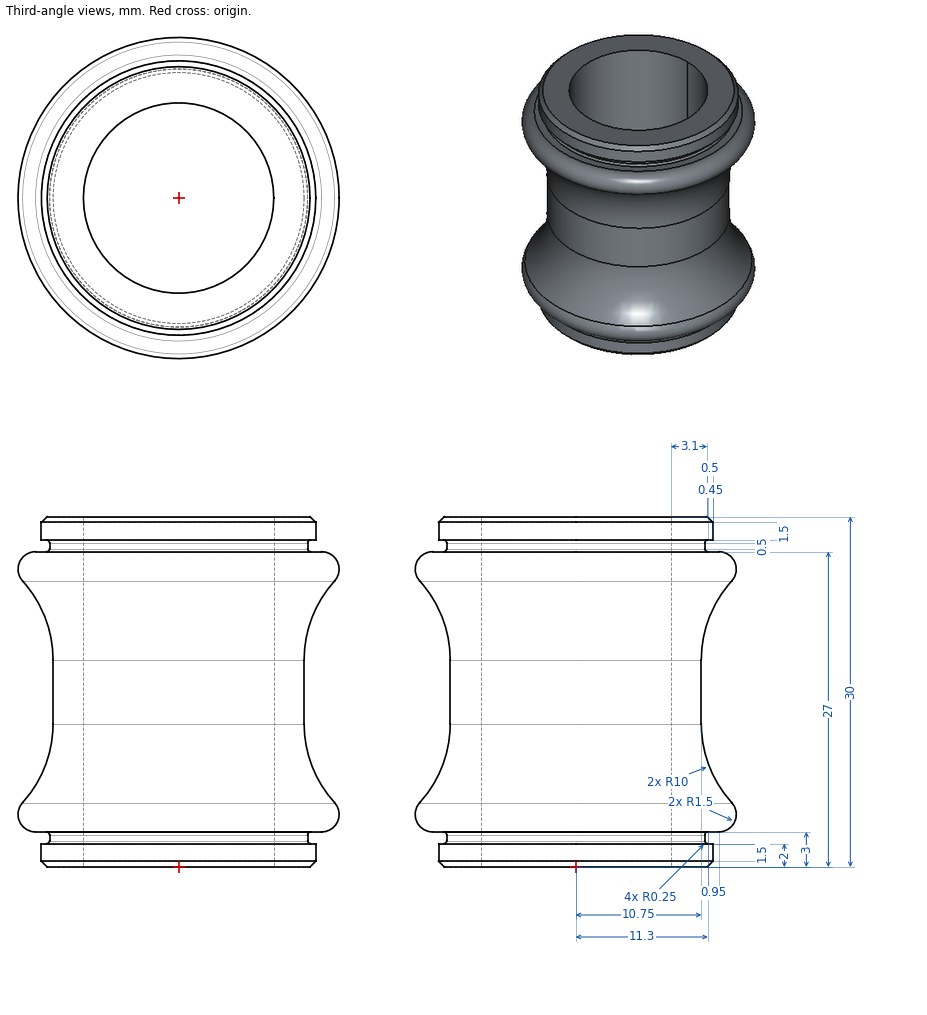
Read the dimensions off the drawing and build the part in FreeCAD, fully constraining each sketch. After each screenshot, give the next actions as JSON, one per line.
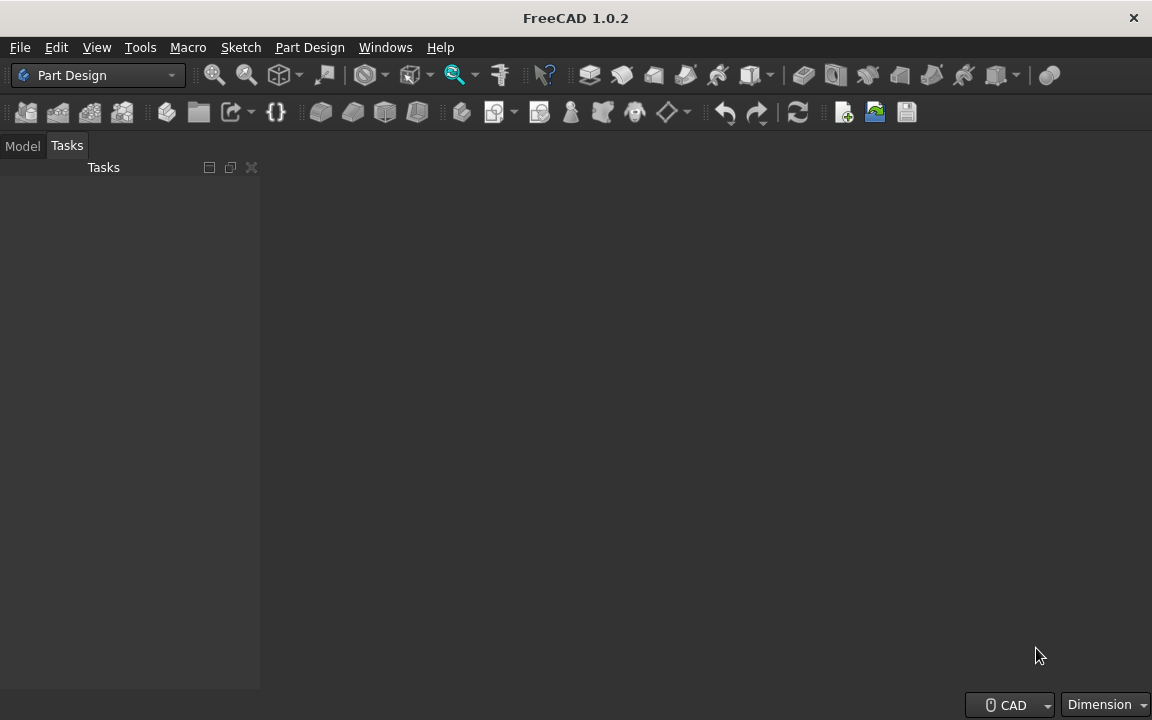
{"action": "left_click", "coordinate": [844, 112]}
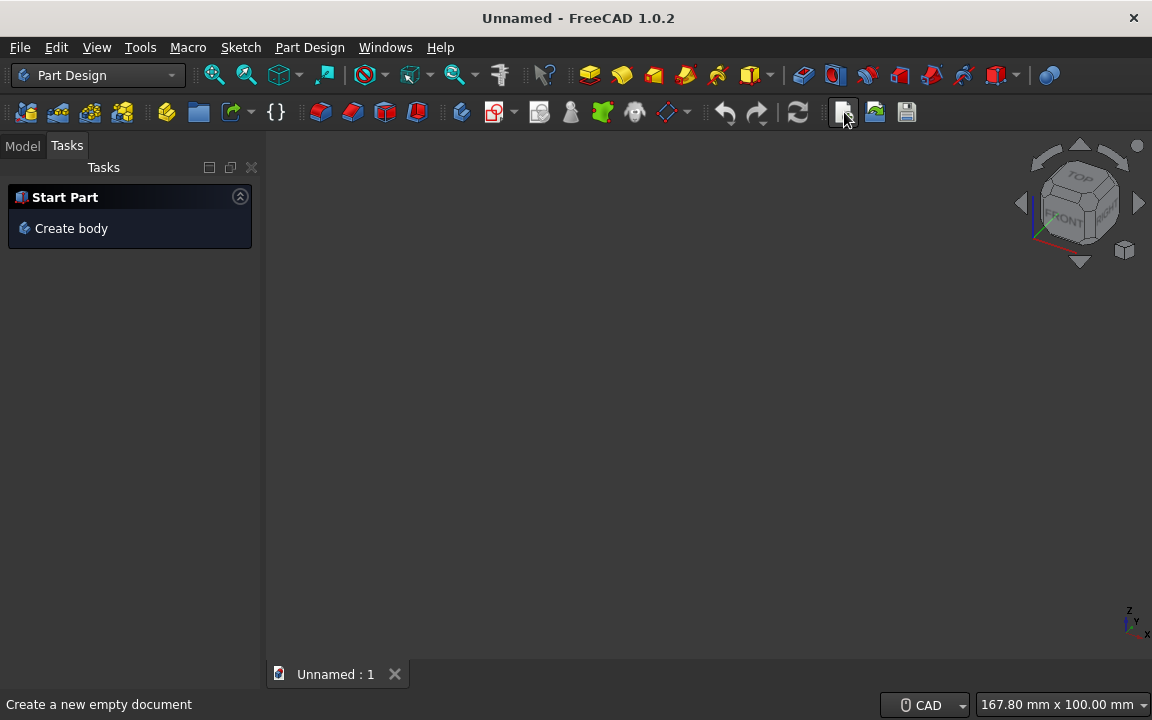
{"action": "left_click", "coordinate": [494, 112]}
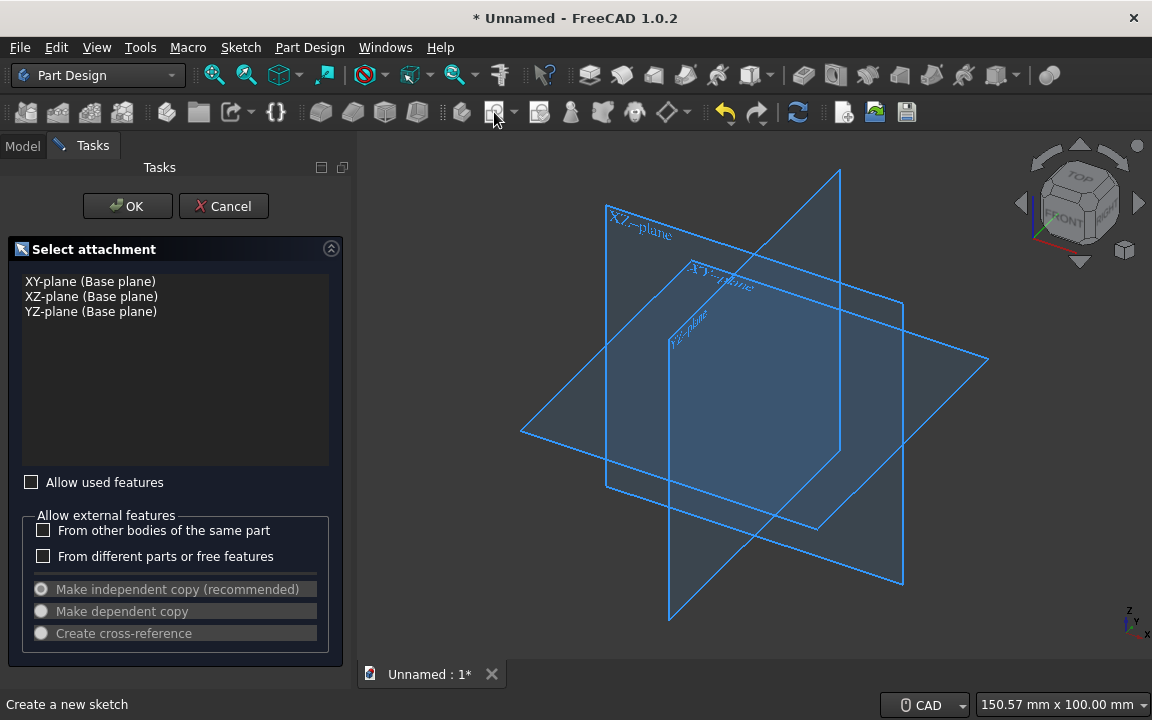
{"action": "left_click", "coordinate": [82, 312]}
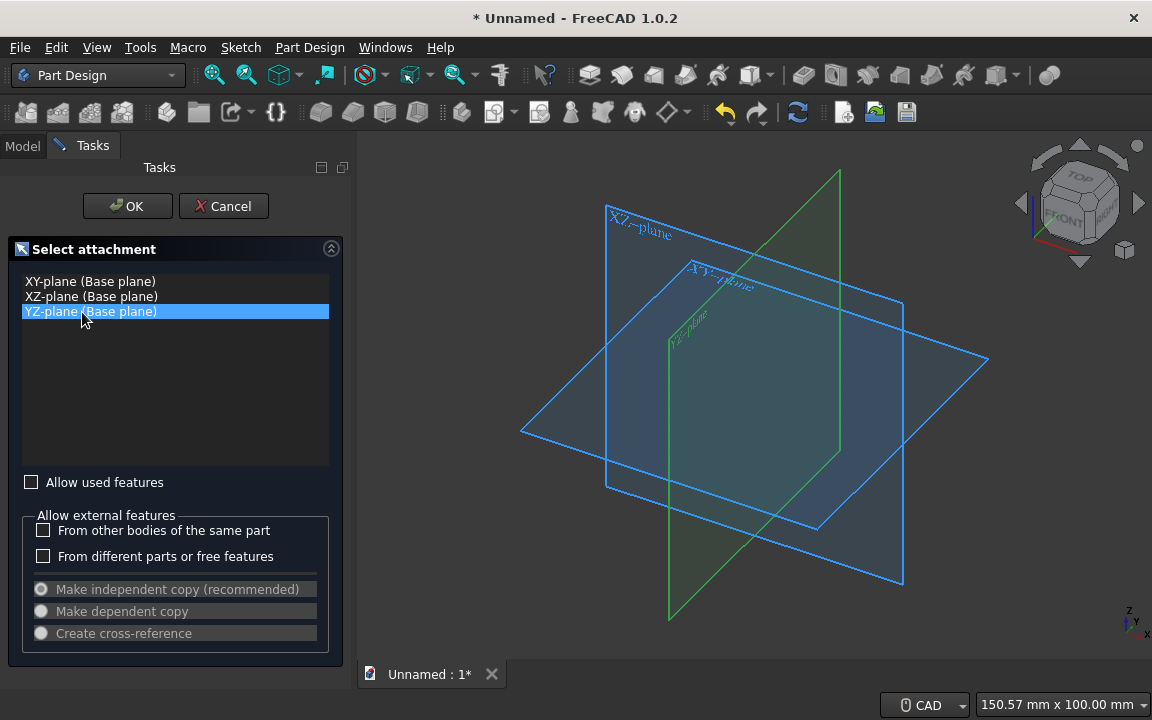
{"action": "left_click", "coordinate": [128, 206]}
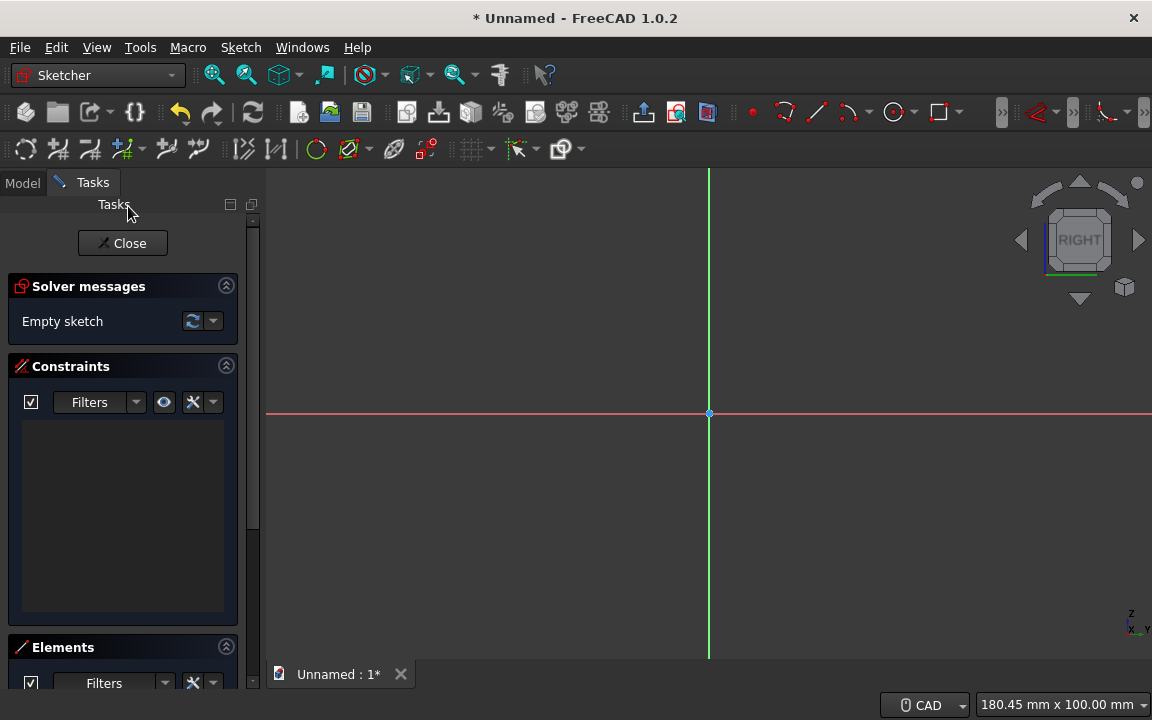
{"action": "scroll", "coordinate": [826, 280], "scroll_direction": "up", "scroll_amount": 4}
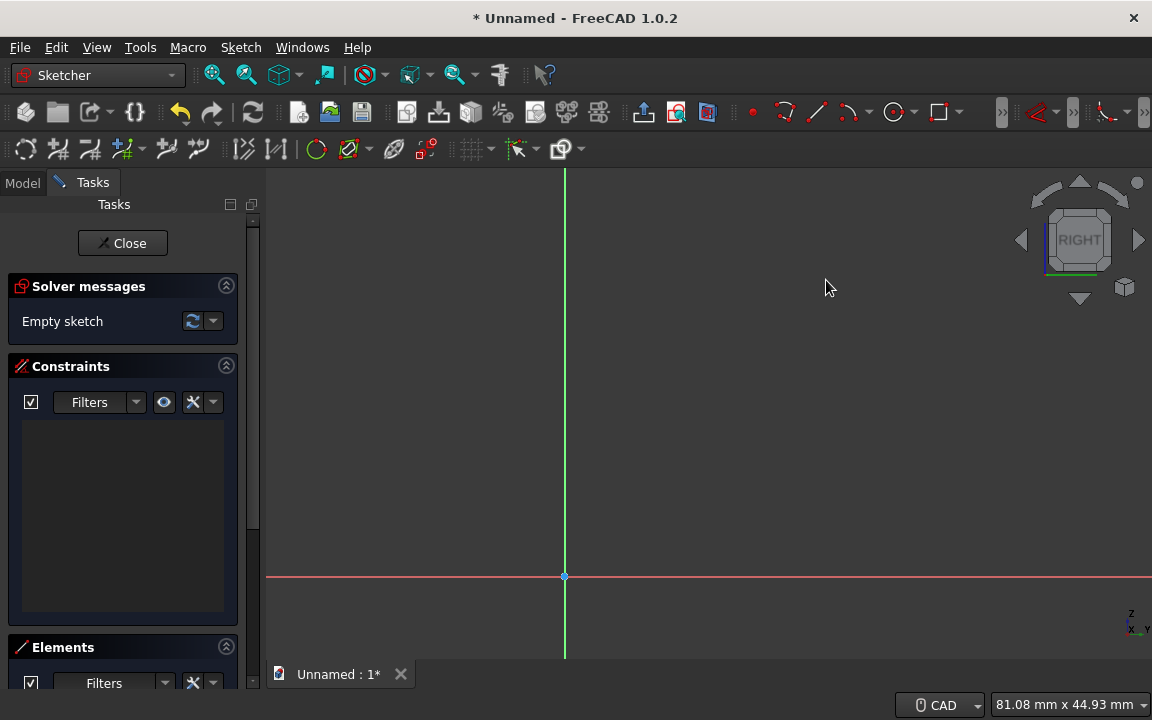
{"action": "left_click", "coordinate": [818, 112]}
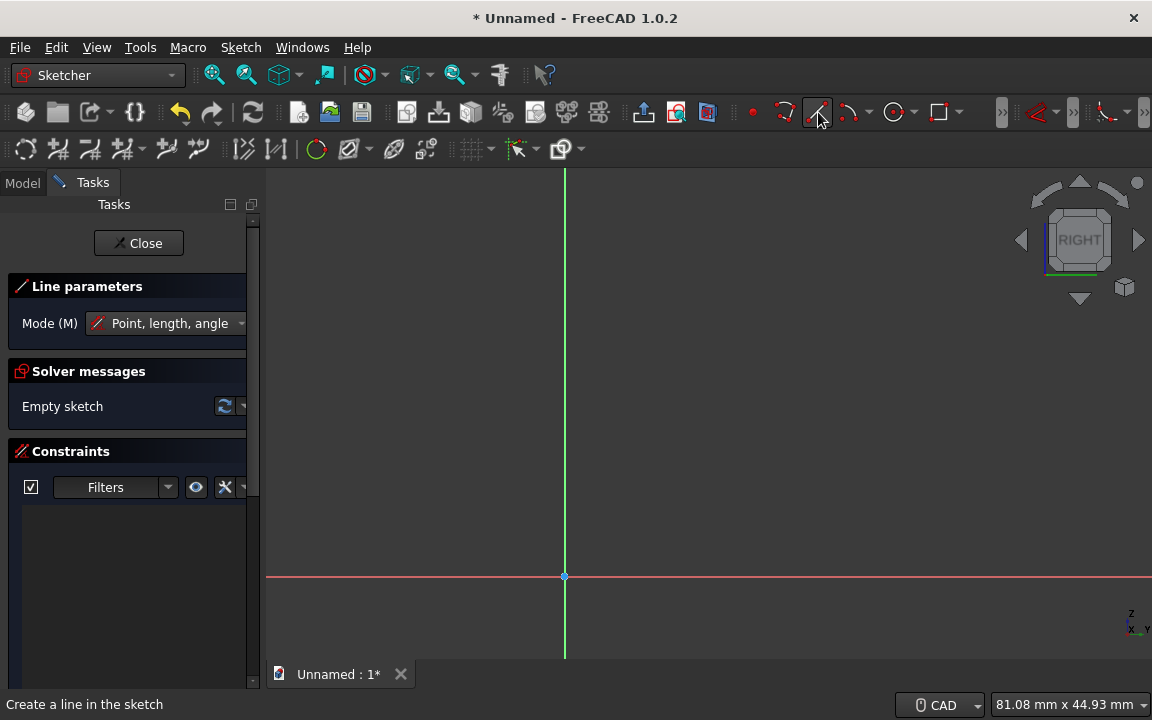
{"action": "left_click", "coordinate": [686, 552]}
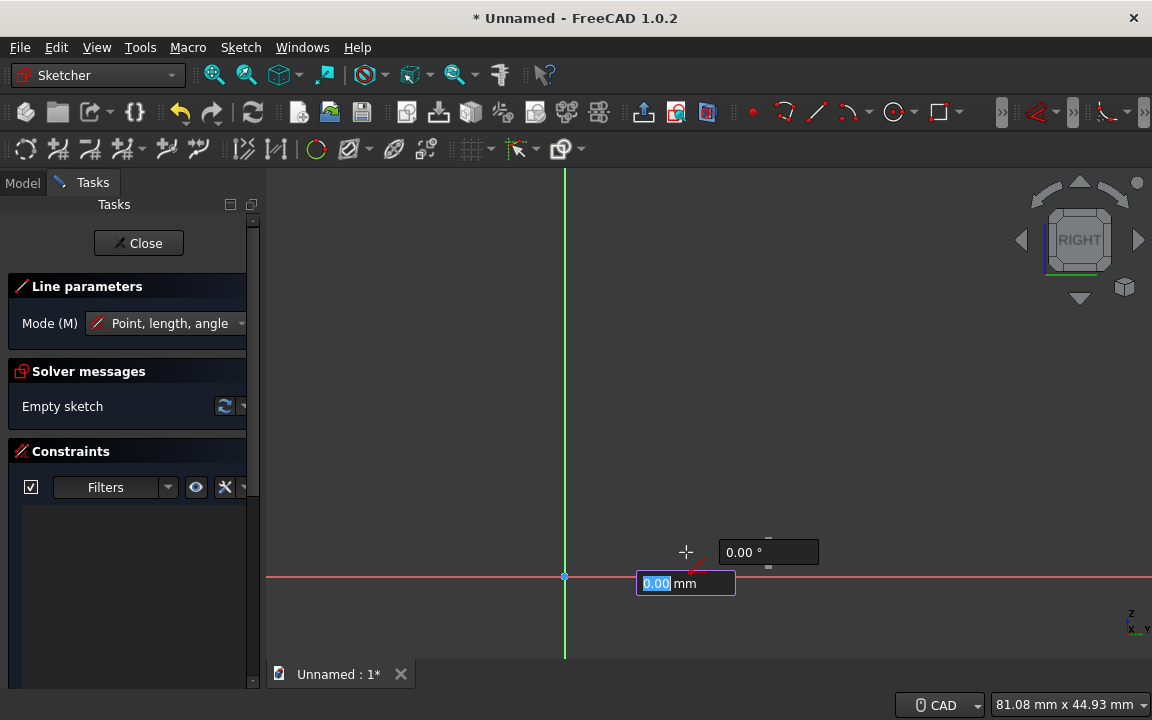
{"action": "scroll", "coordinate": [686, 547], "scroll_direction": "up", "scroll_amount": 6}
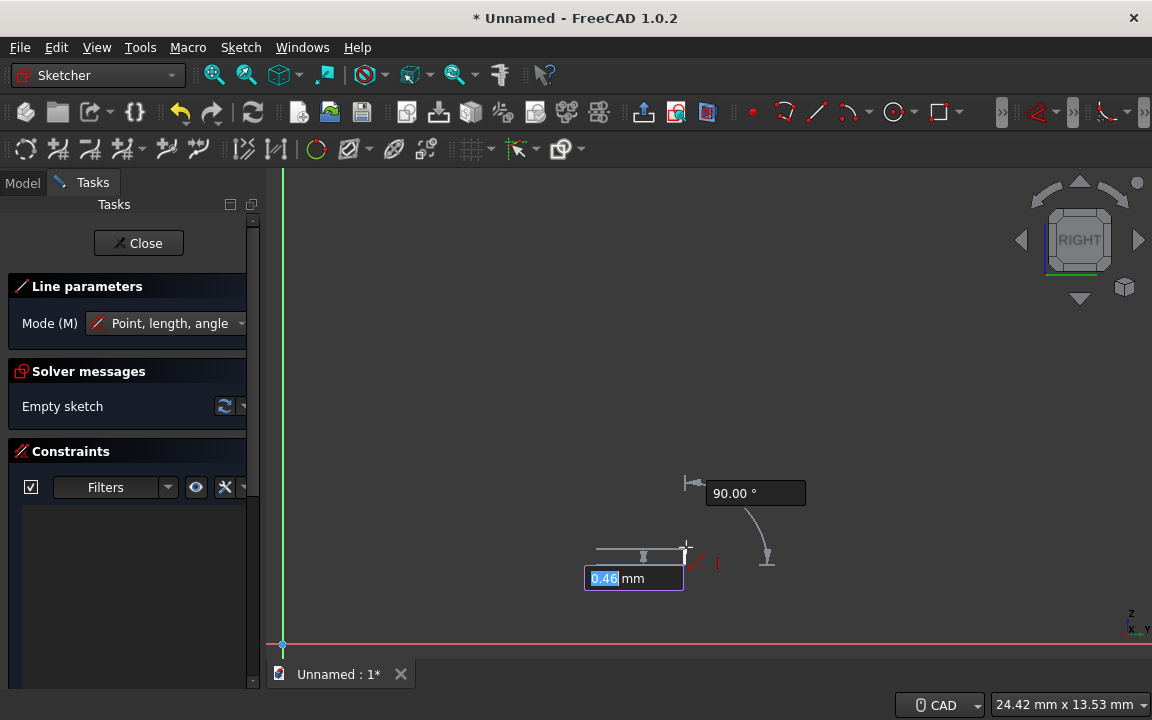
{"action": "left_click", "coordinate": [685, 544]}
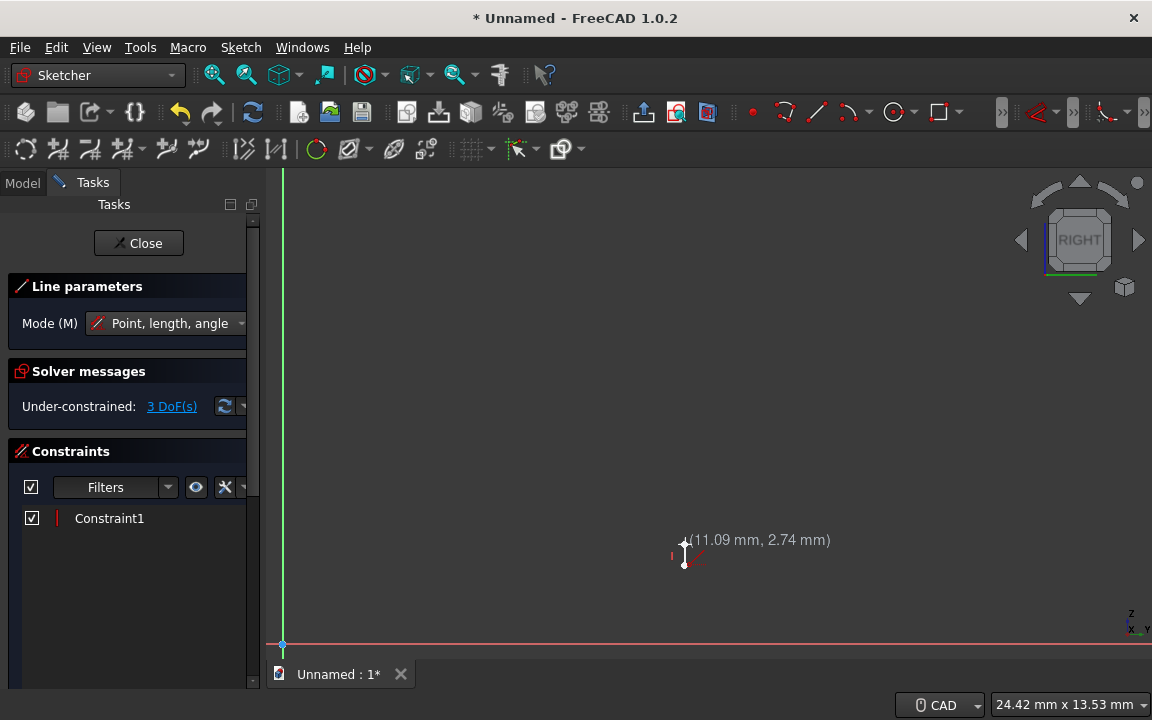
{"action": "scroll", "coordinate": [693, 535], "scroll_direction": "up", "scroll_amount": 2}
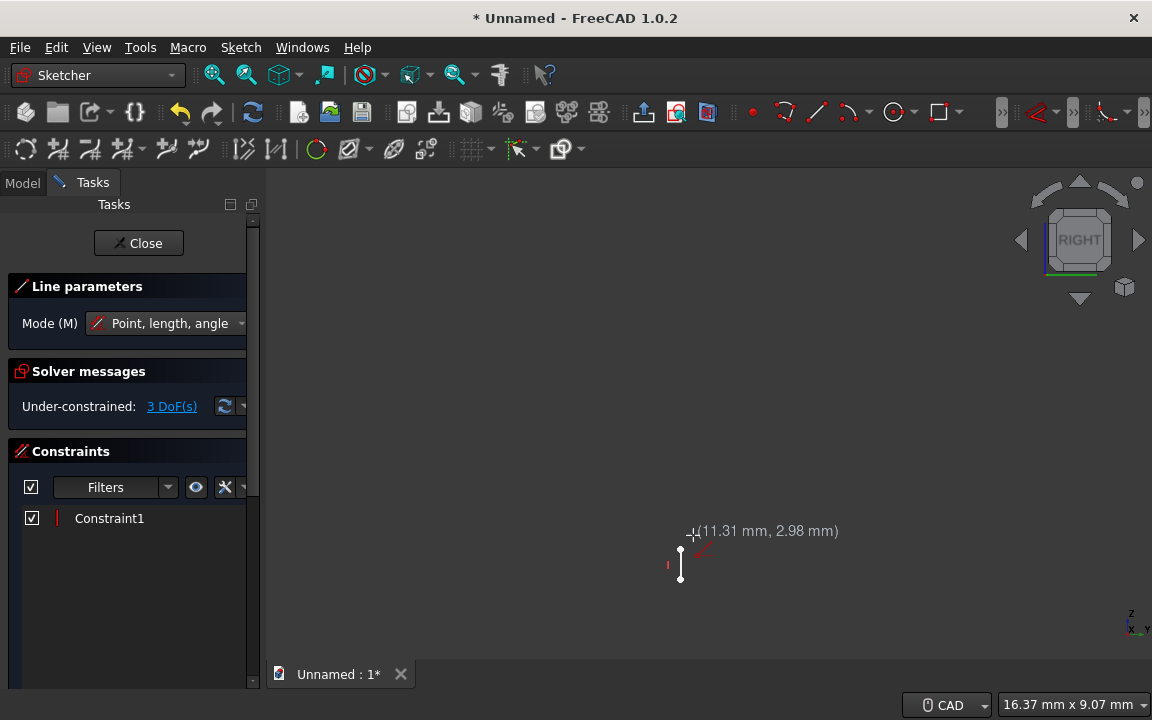
{"action": "left_click", "coordinate": [692, 535]}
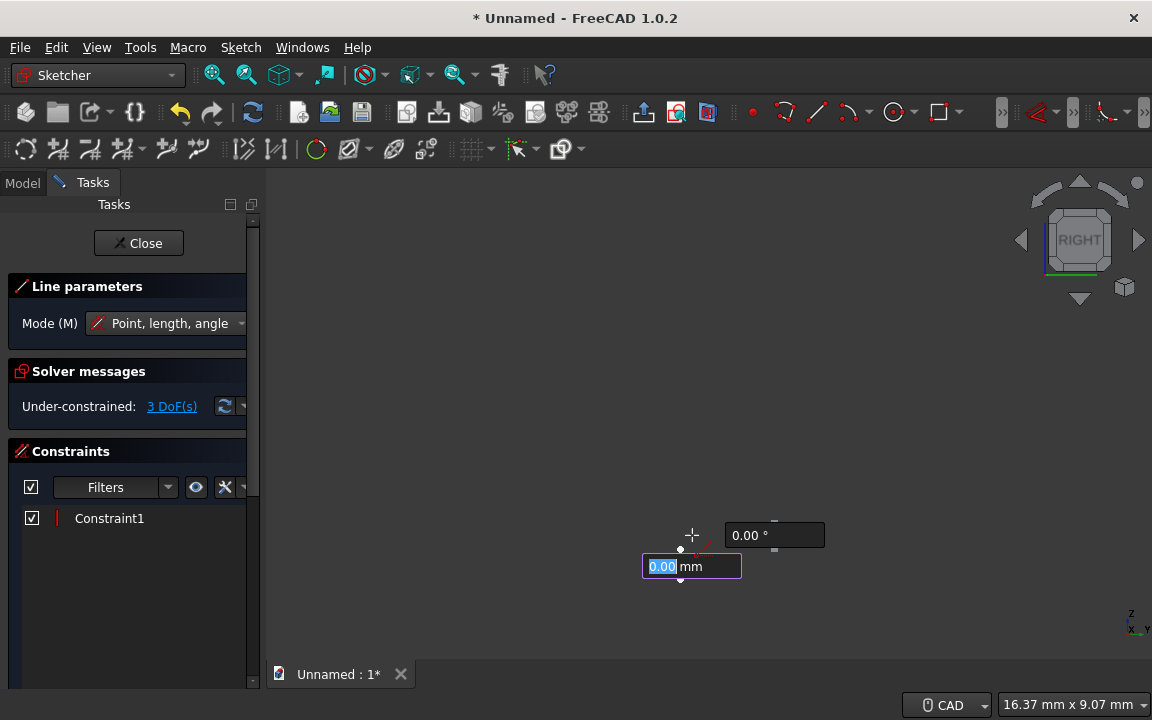
{"action": "scroll", "coordinate": [689, 547], "scroll_direction": "down", "scroll_amount": 8}